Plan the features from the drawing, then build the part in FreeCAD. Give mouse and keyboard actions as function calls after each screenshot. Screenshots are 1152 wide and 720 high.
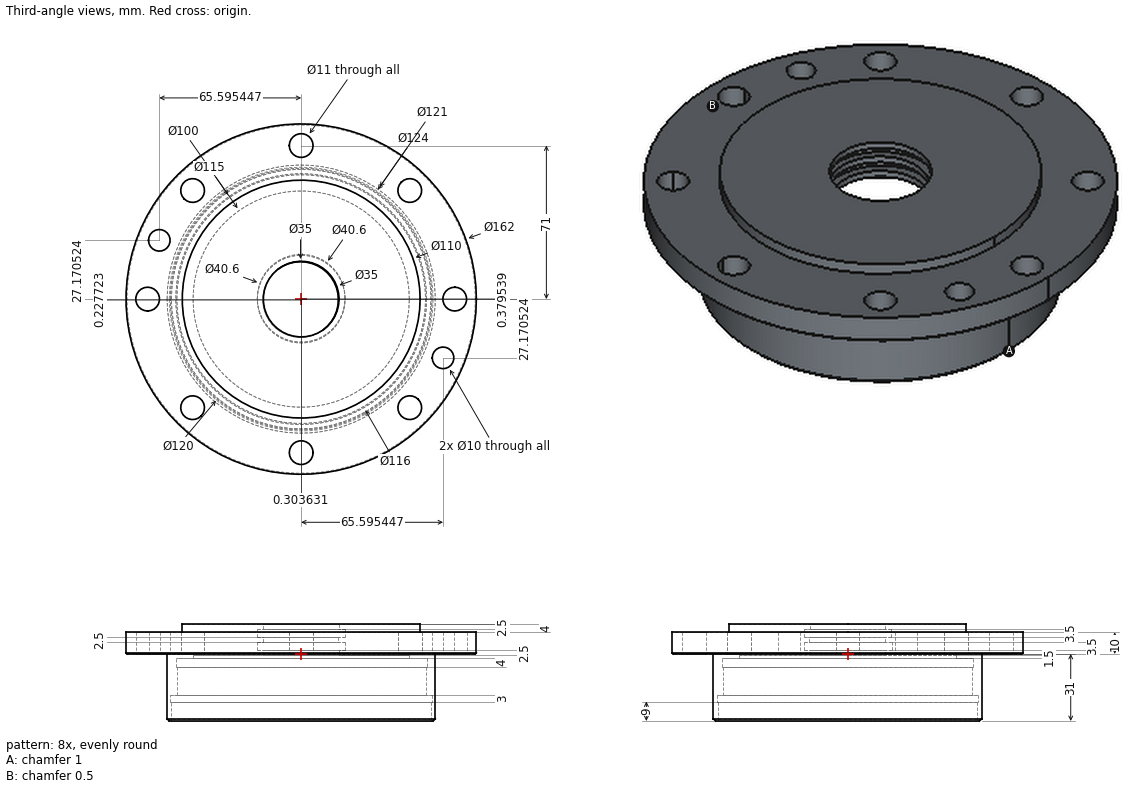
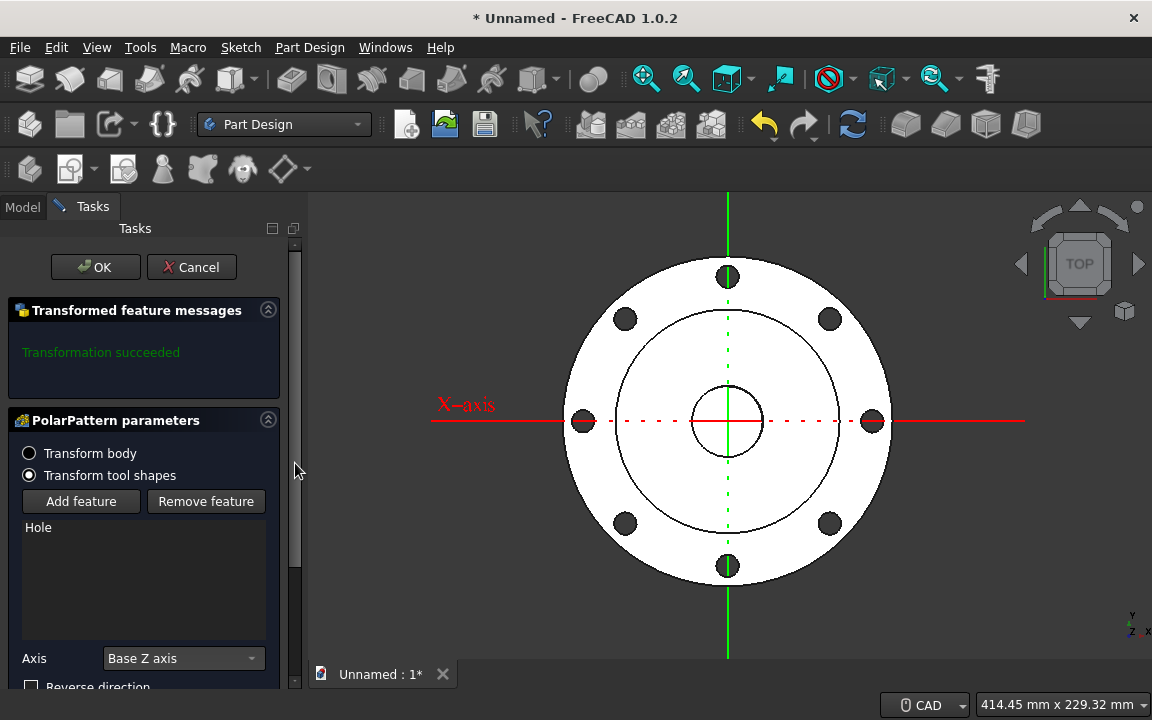
click(96, 267)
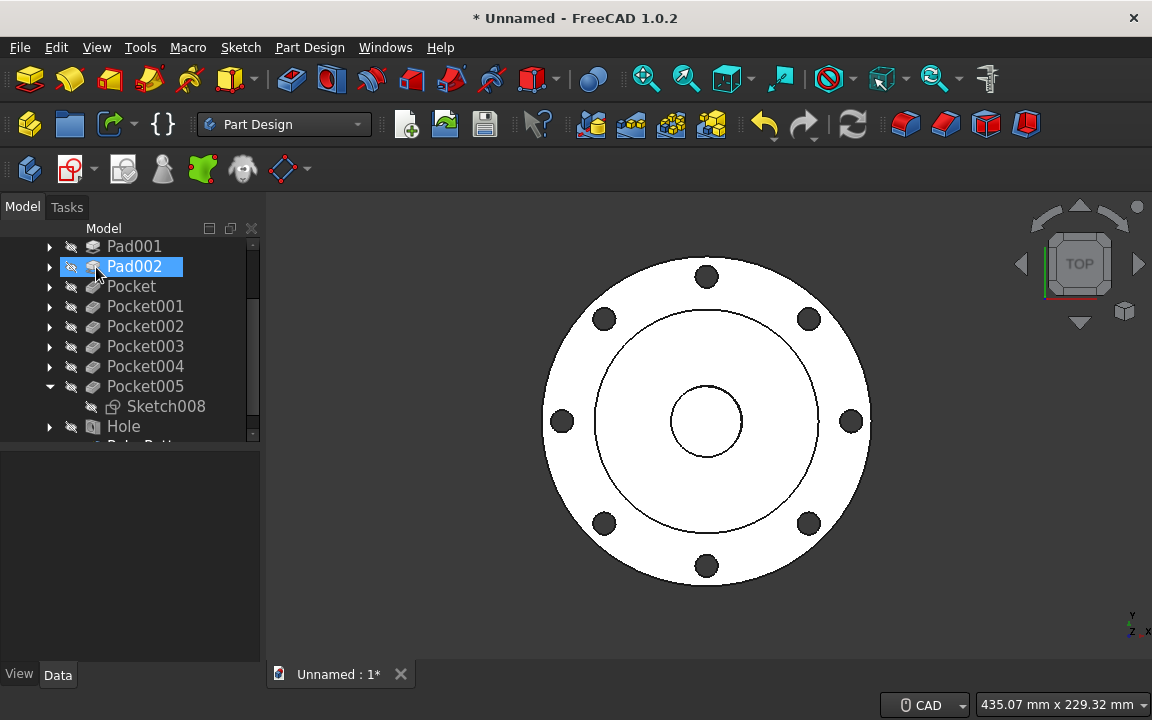
click(848, 467)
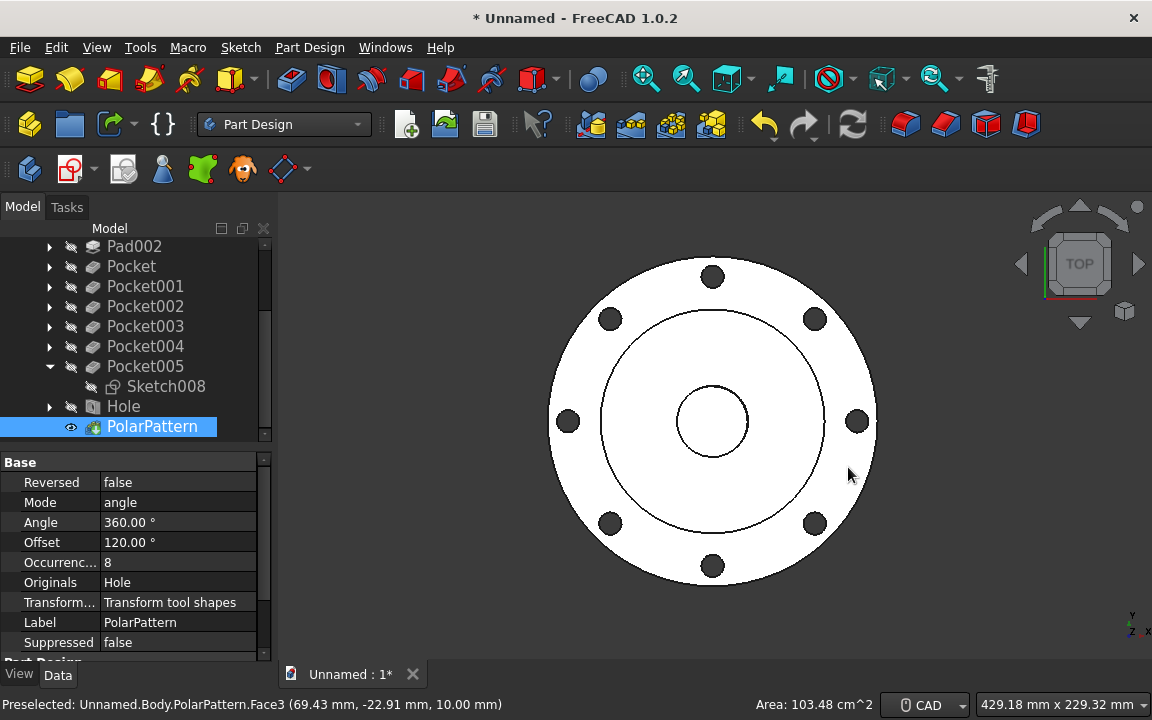
click(70, 170)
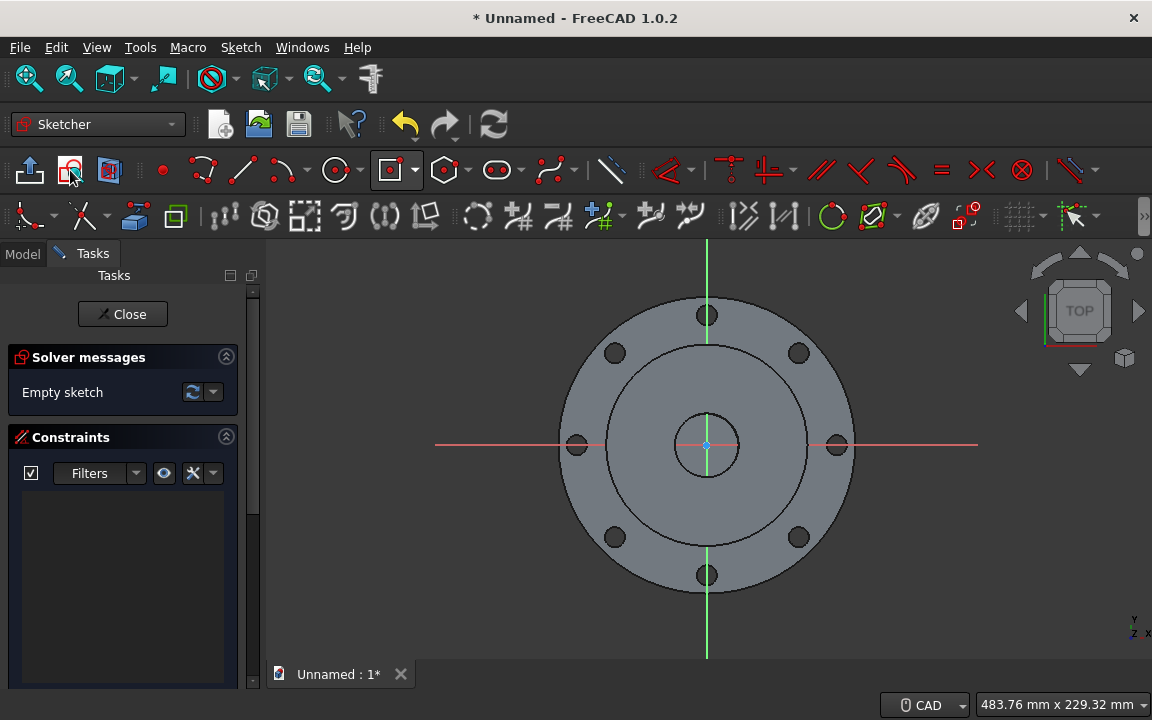
click(110, 170)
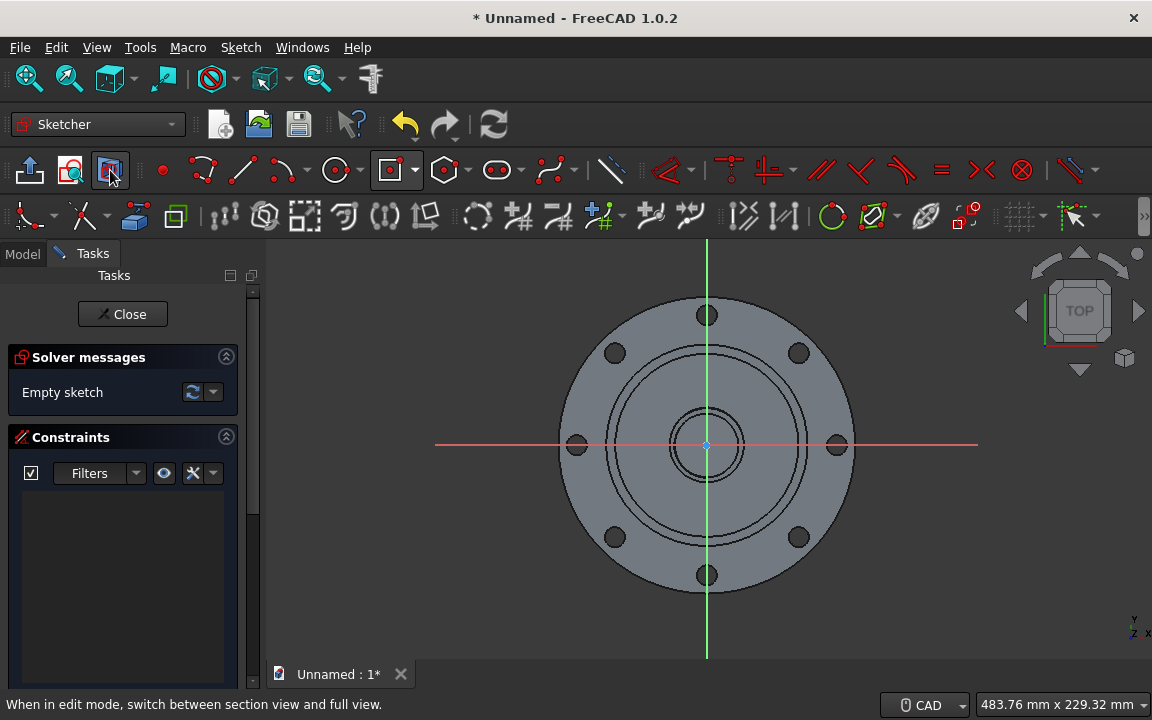
scroll(788, 441, up, 3)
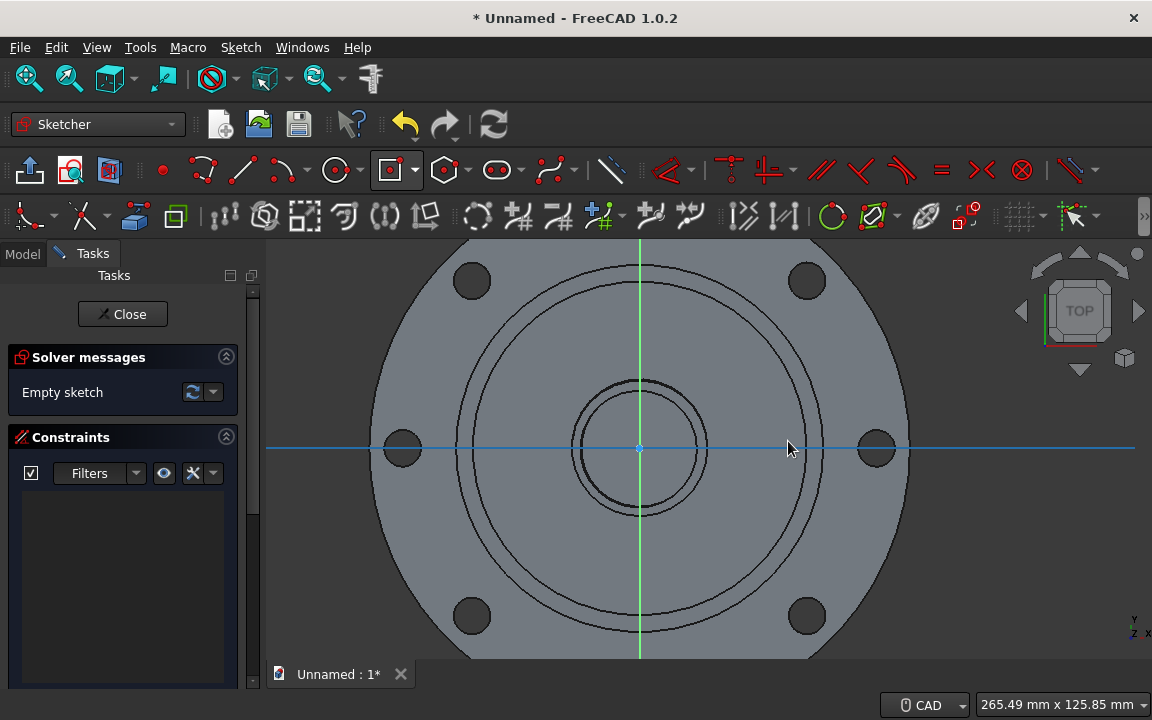
click(336, 170)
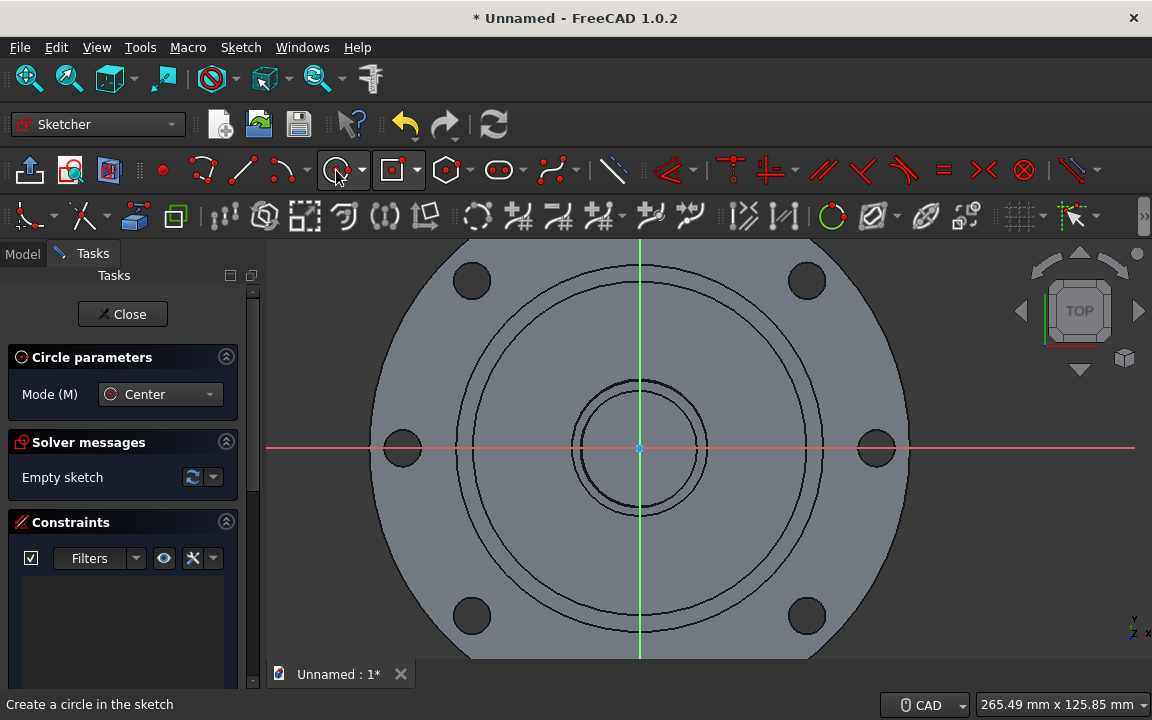
scroll(859, 539, up, 2)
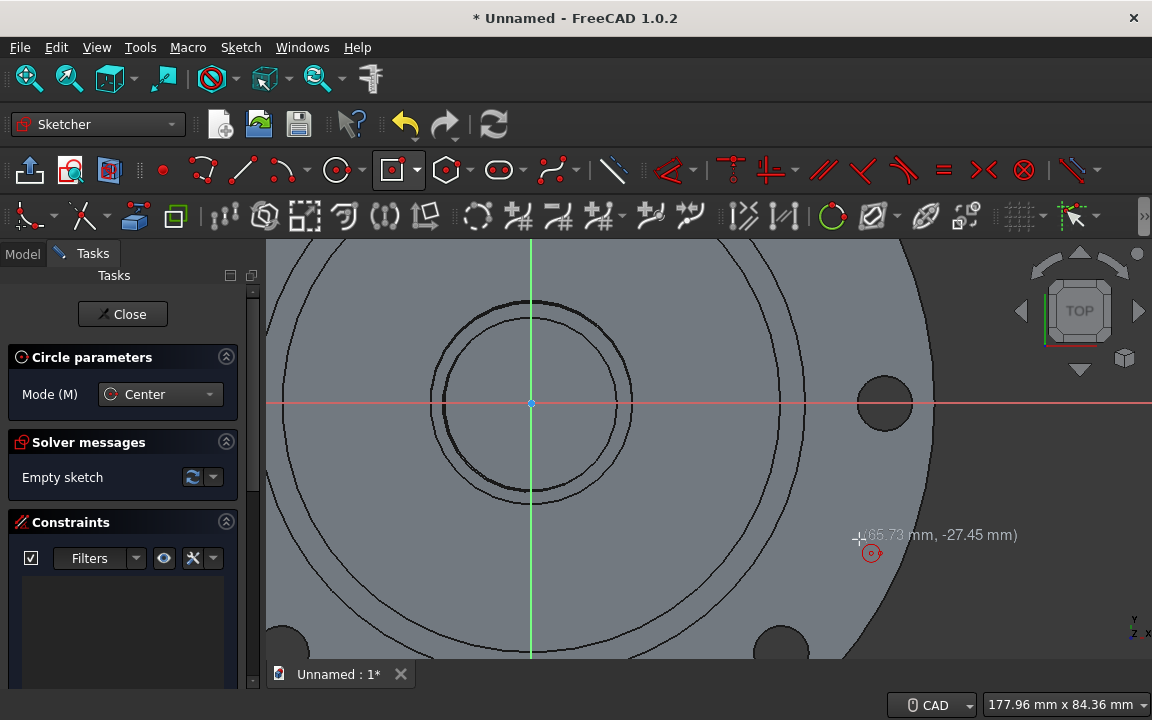
click(858, 539)
click(876, 521)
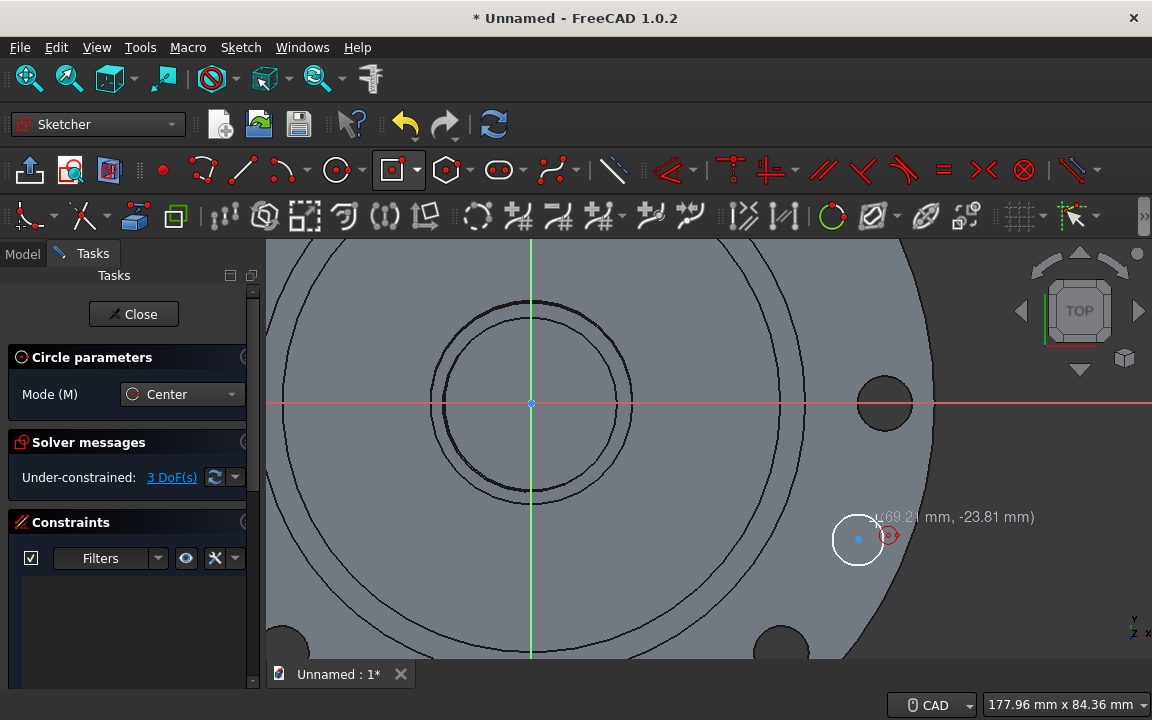
scroll(862, 542, down, 2)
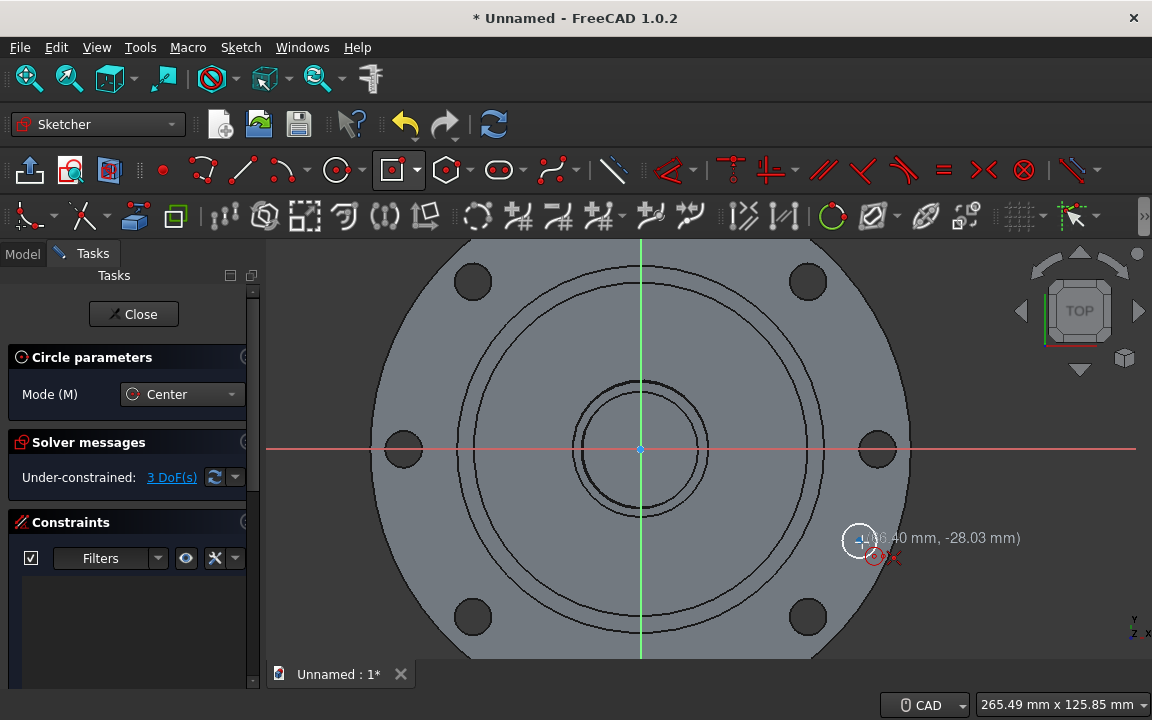
scroll(422, 359, up, 2)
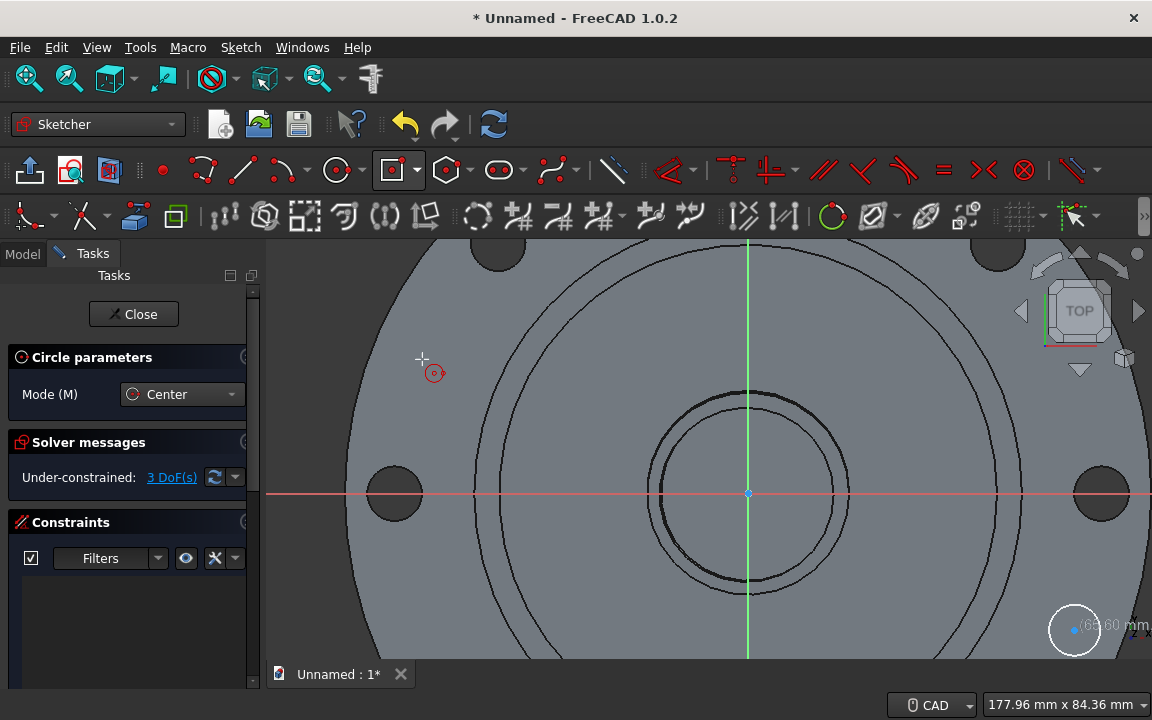
click(422, 358)
click(439, 341)
key(Escape)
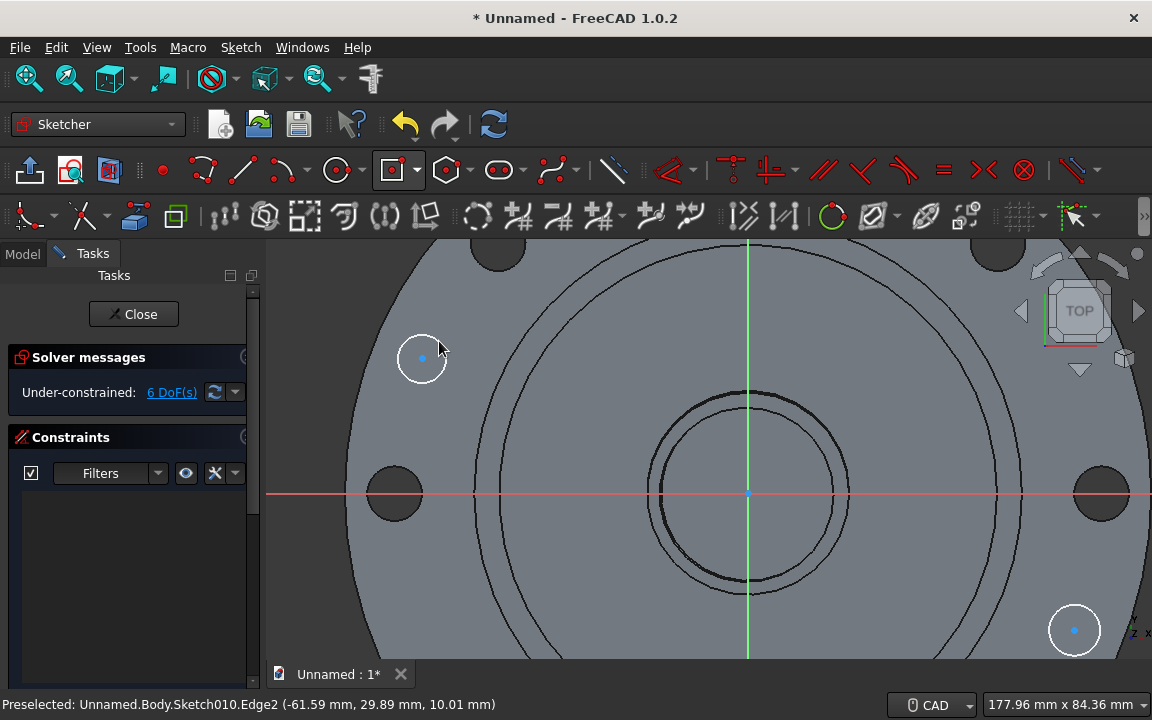
scroll(422, 358, down, 2)